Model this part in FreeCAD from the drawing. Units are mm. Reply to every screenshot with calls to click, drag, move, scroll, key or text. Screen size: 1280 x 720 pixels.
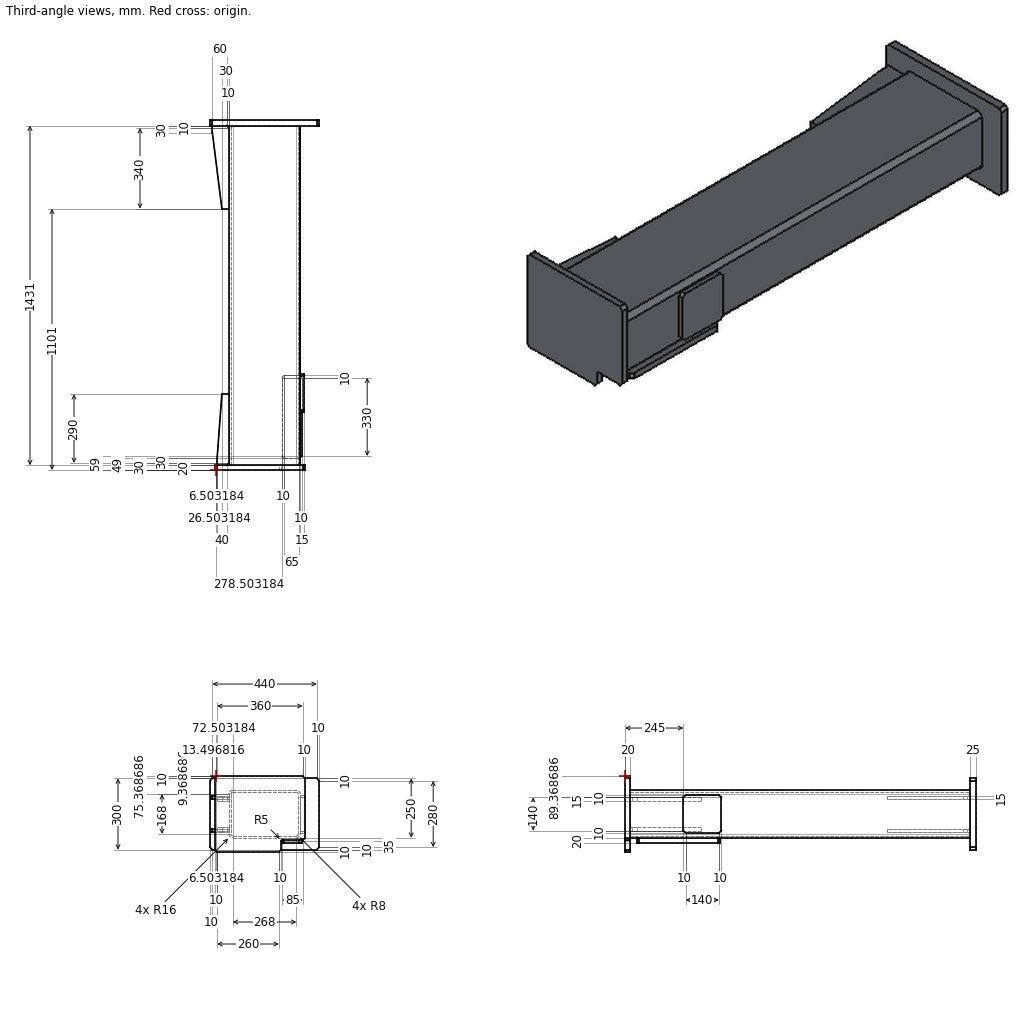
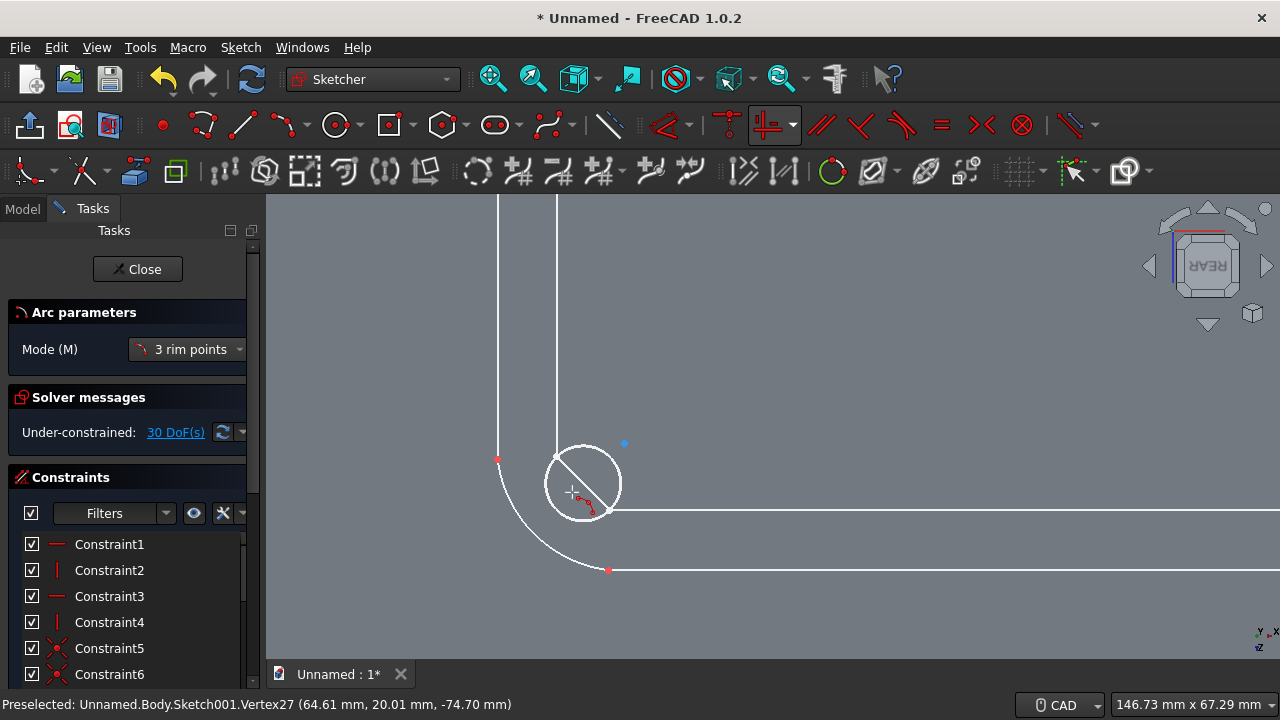
click(572, 491)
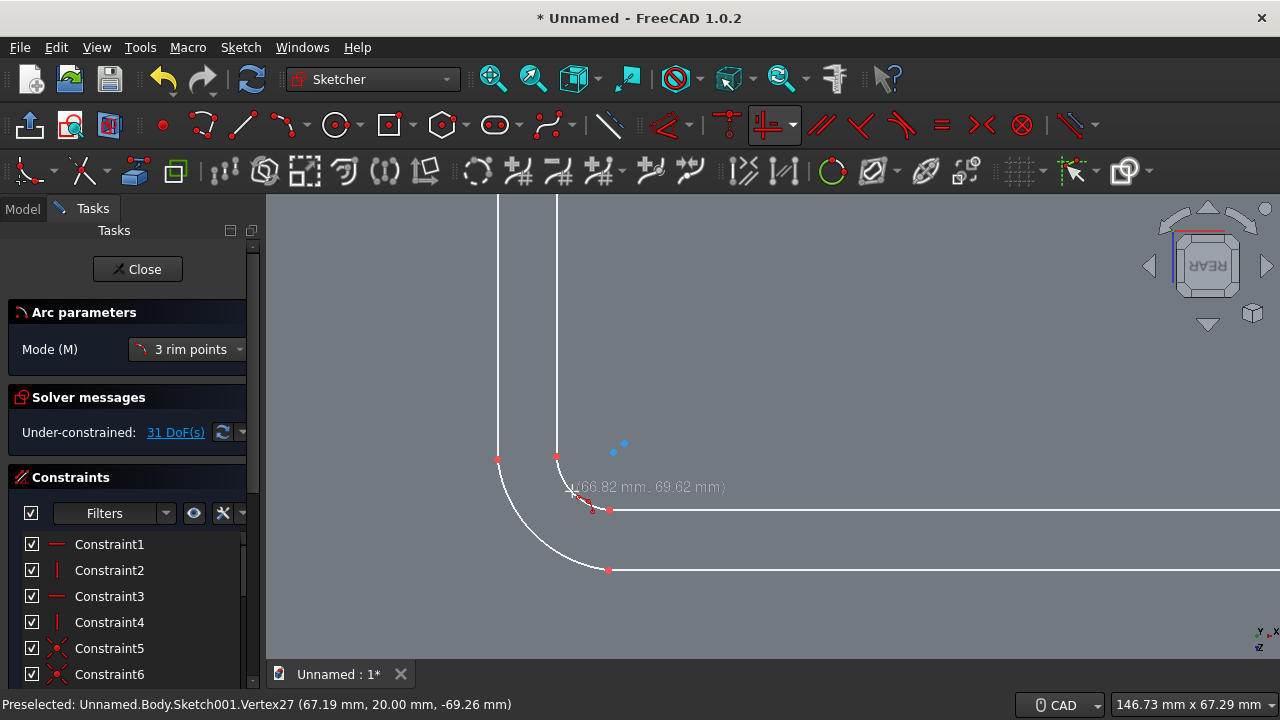
scroll(578, 496, down, 9)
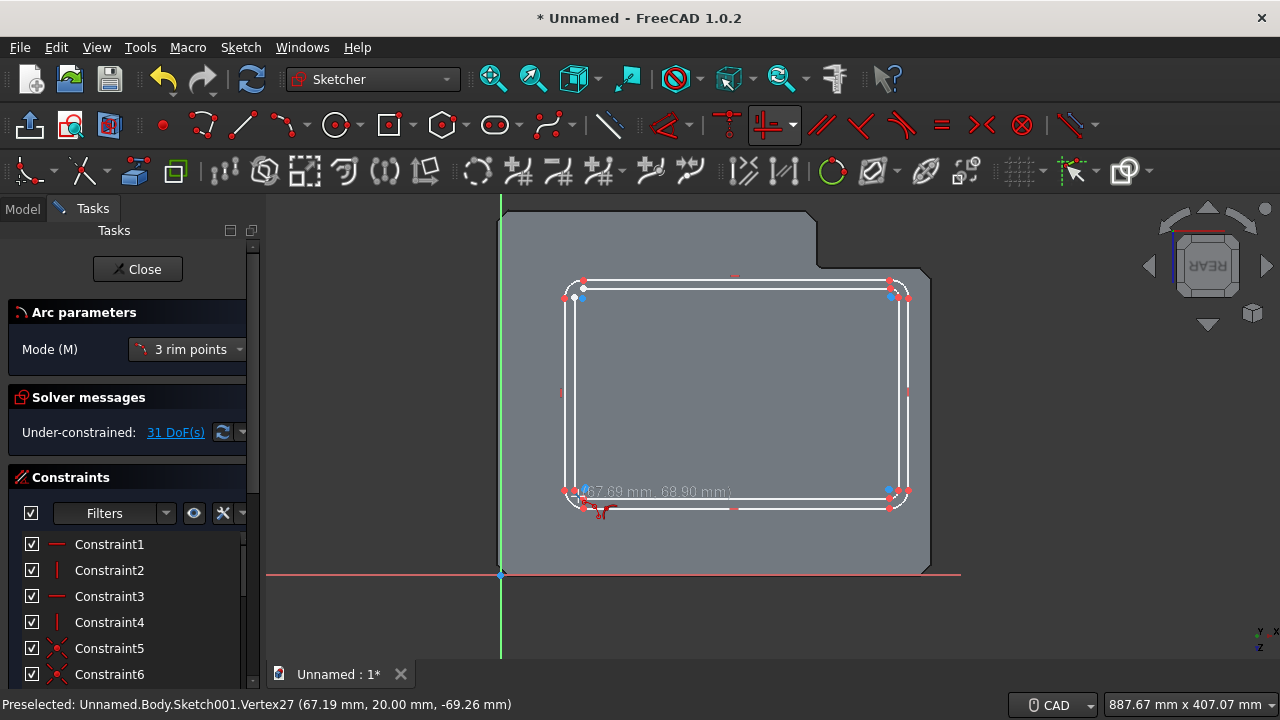
scroll(575, 297, up, 3)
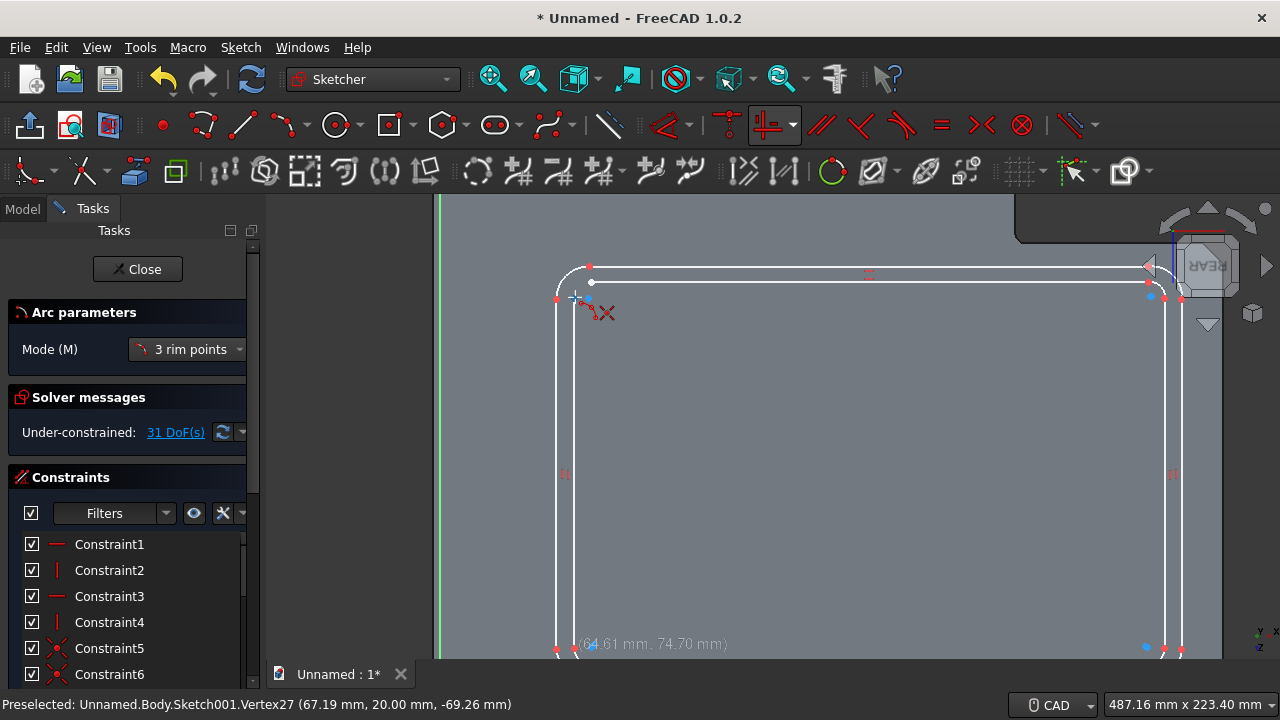
click(574, 299)
click(591, 282)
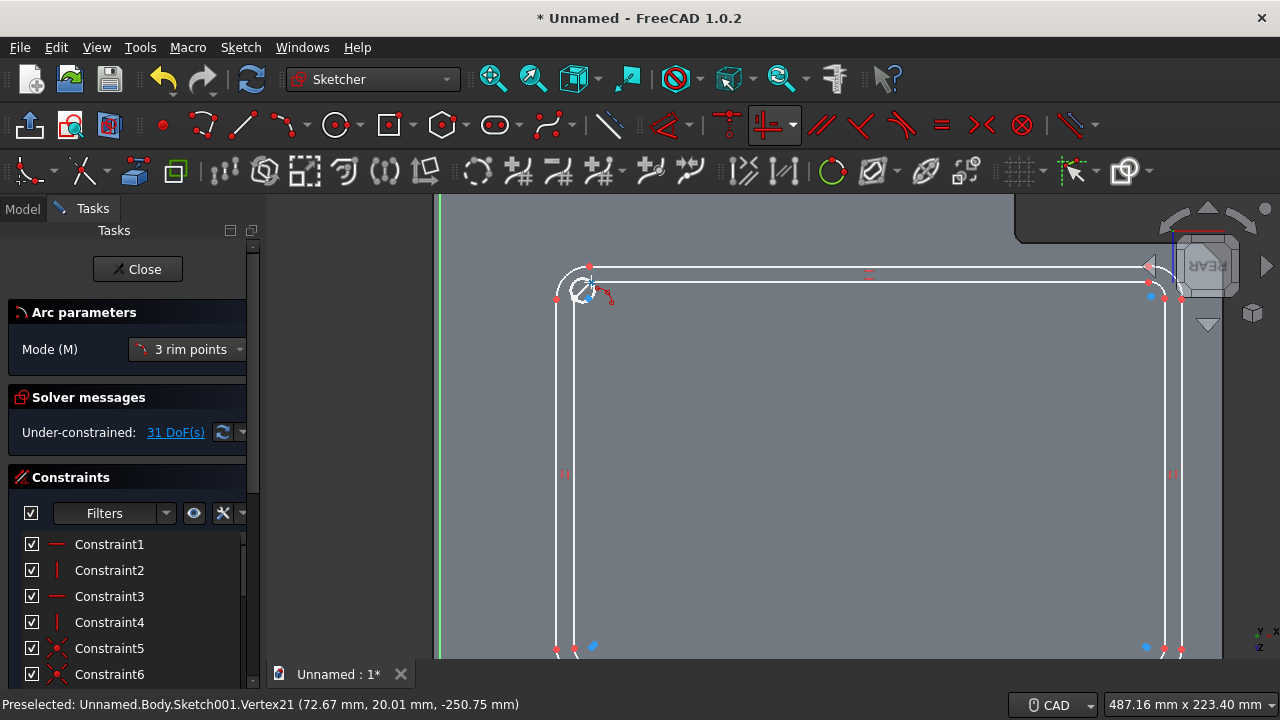
scroll(579, 286, up, 6)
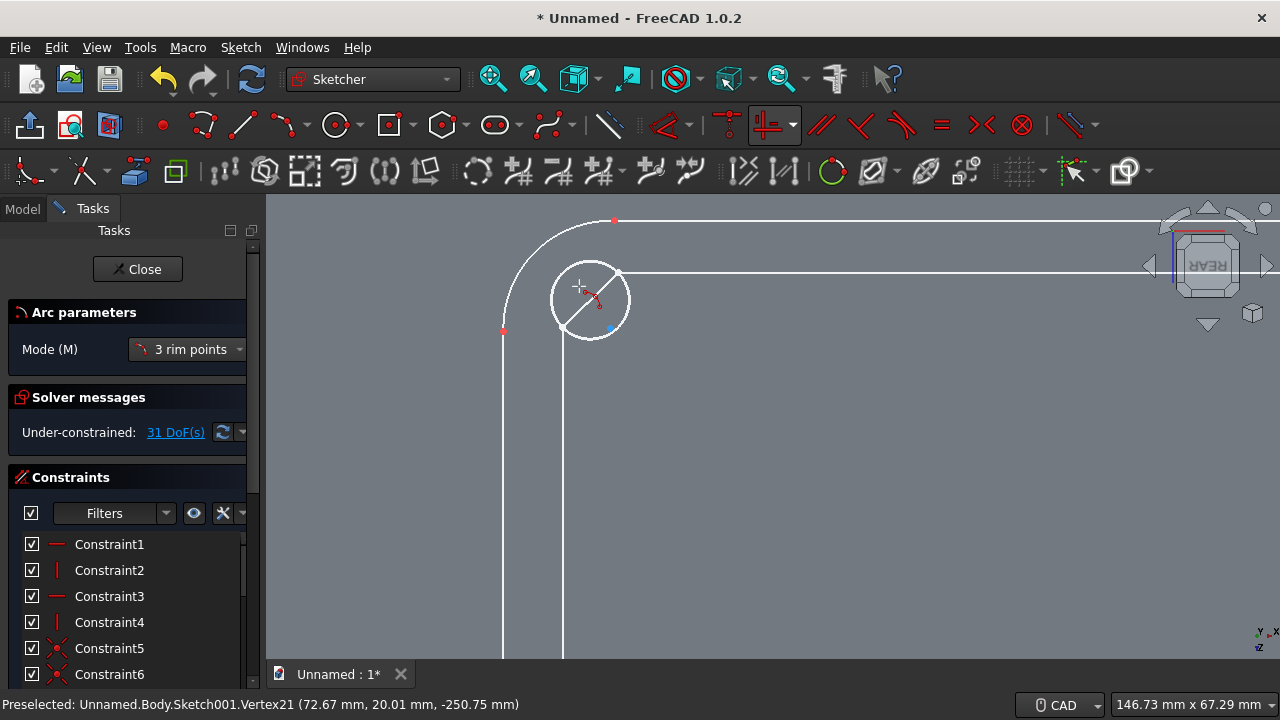
click(578, 285)
key(Escape)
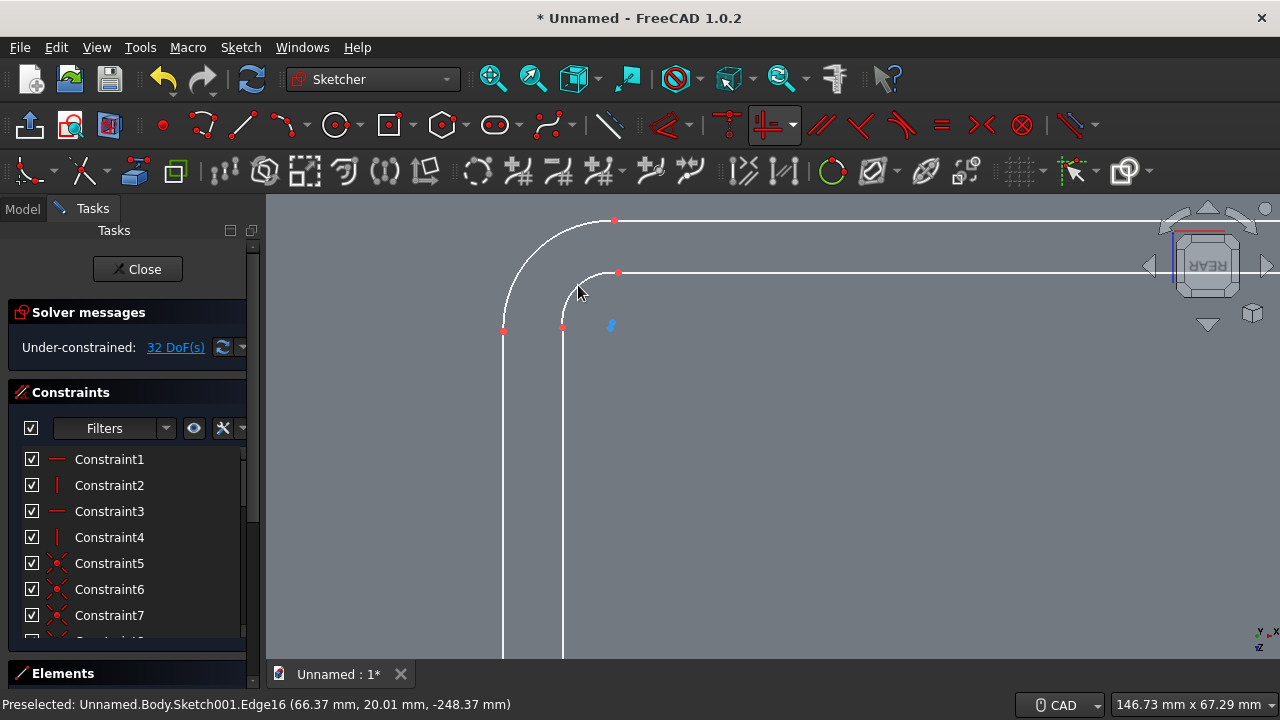
scroll(577, 291, down, 9)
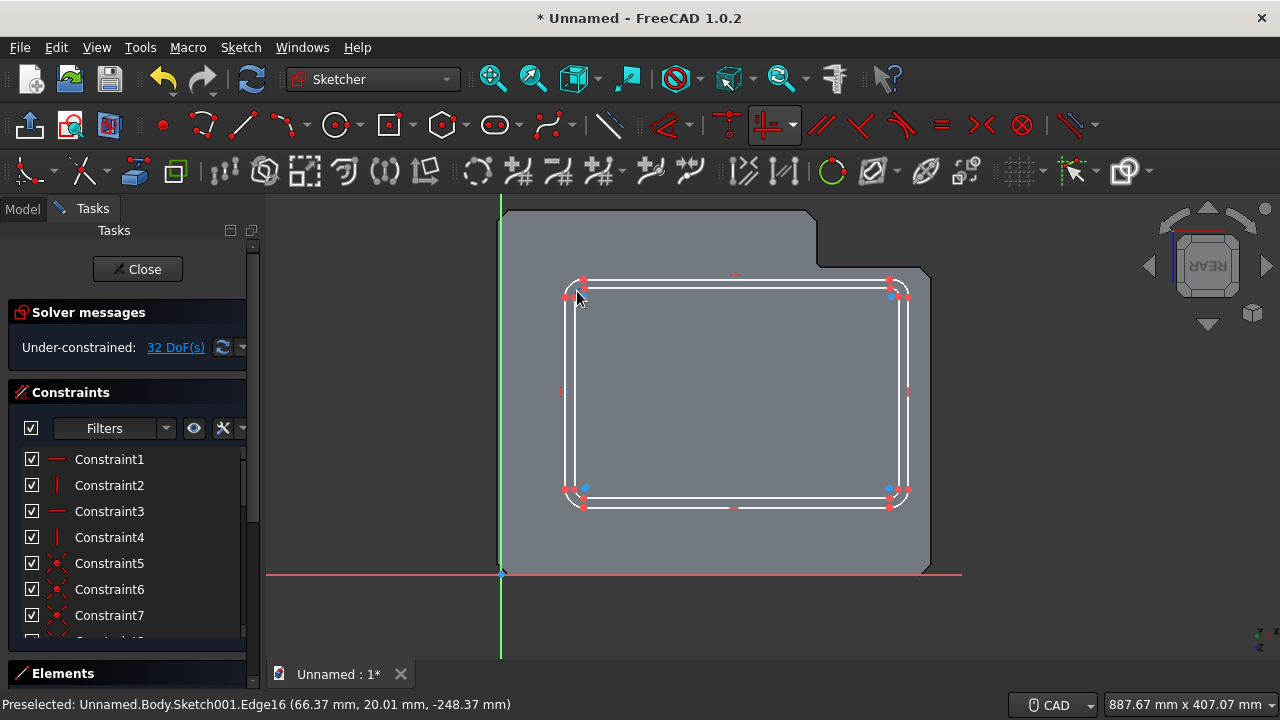
scroll(798, 280, up, 3)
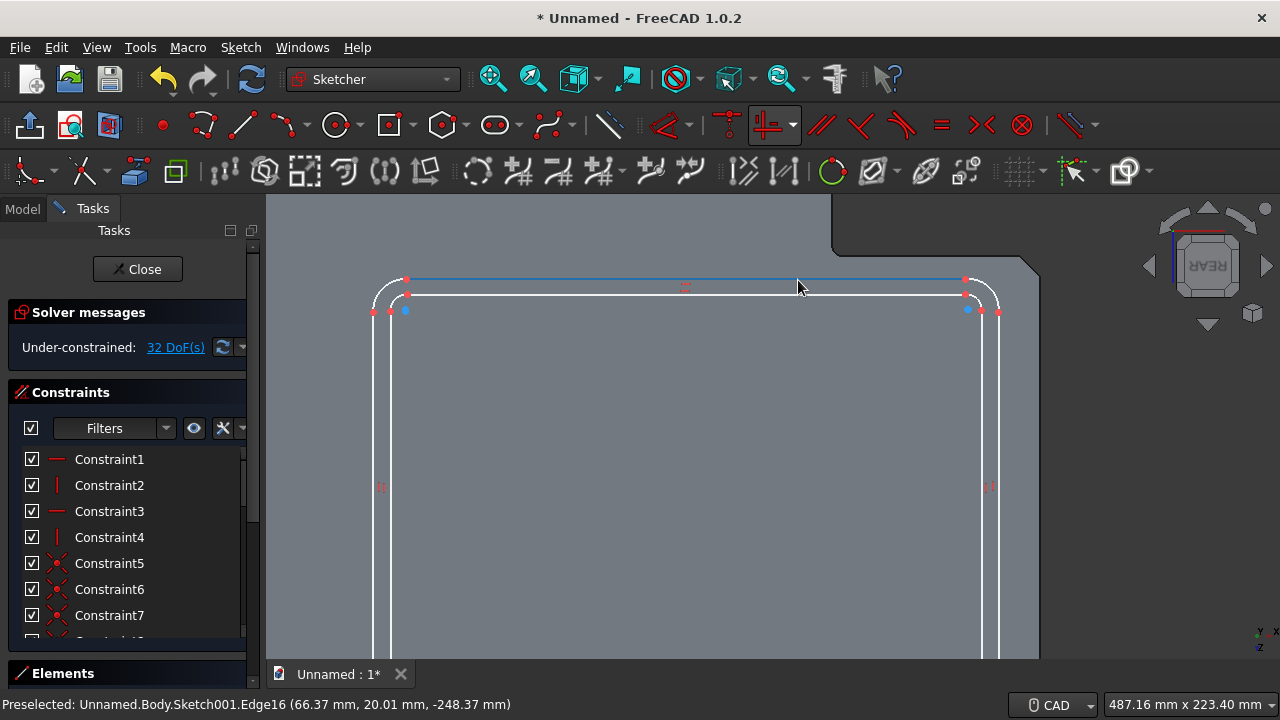
click(798, 279)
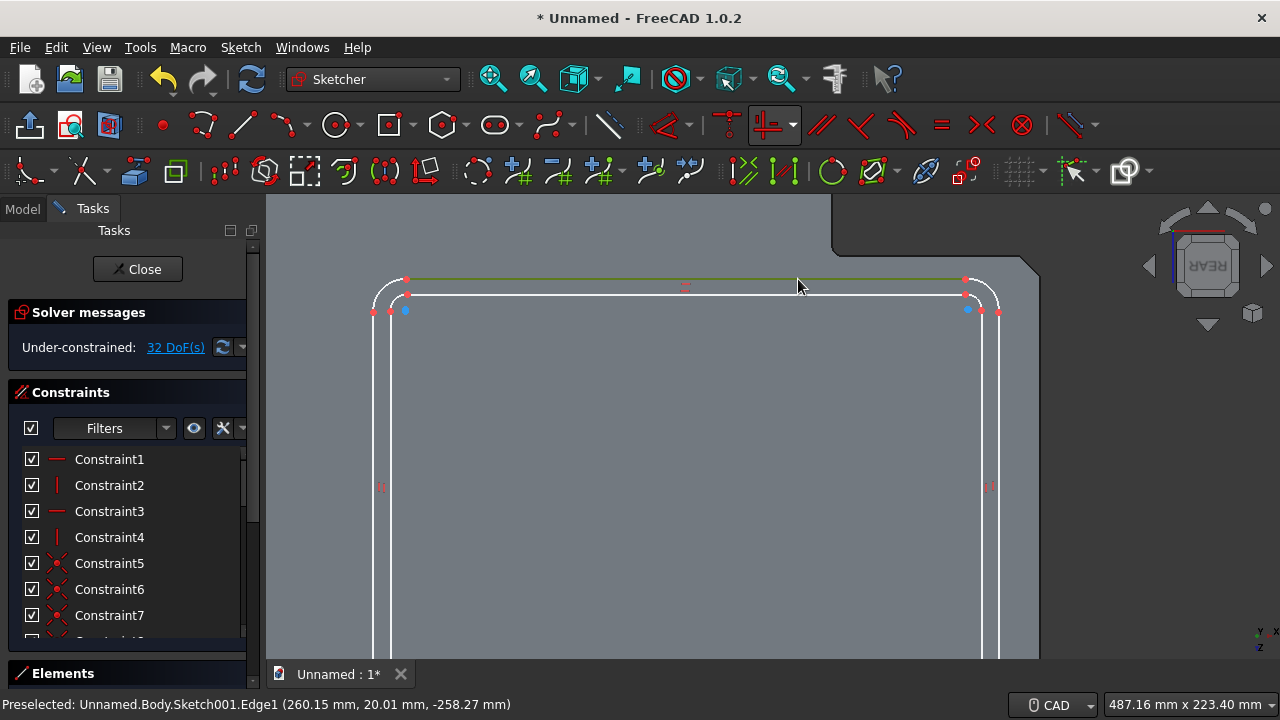
click(391, 282)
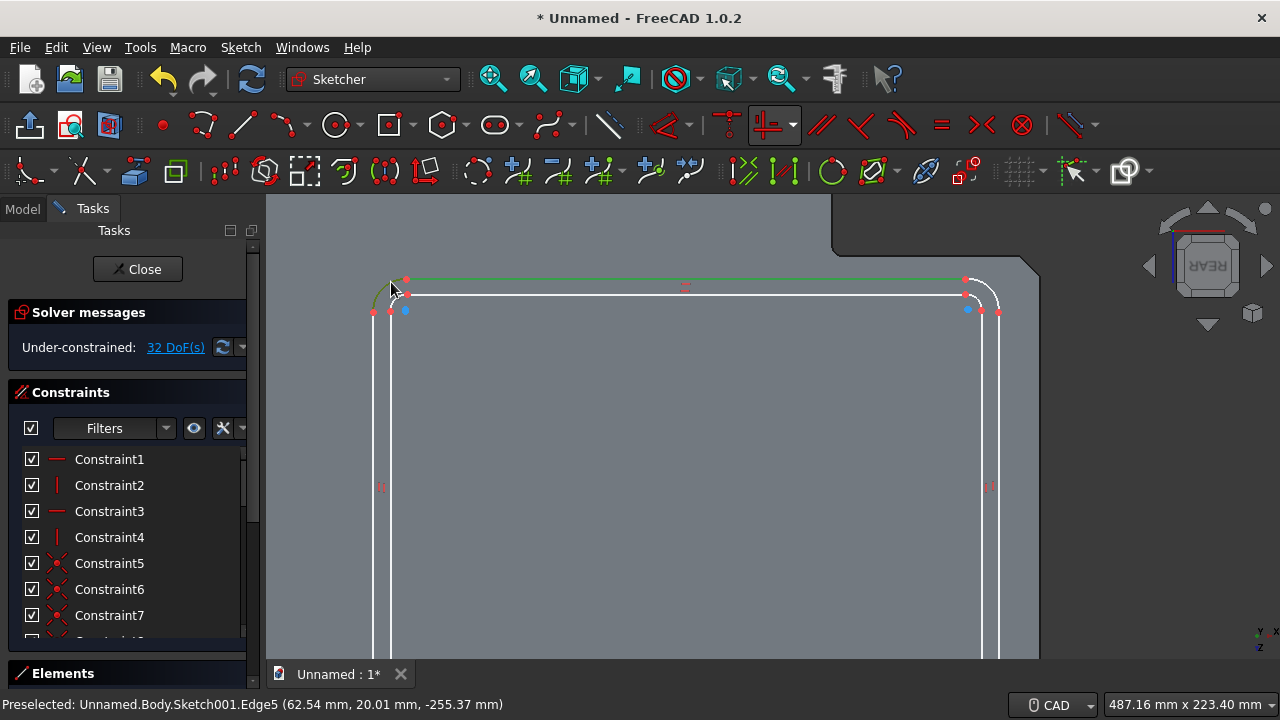
click(902, 126)